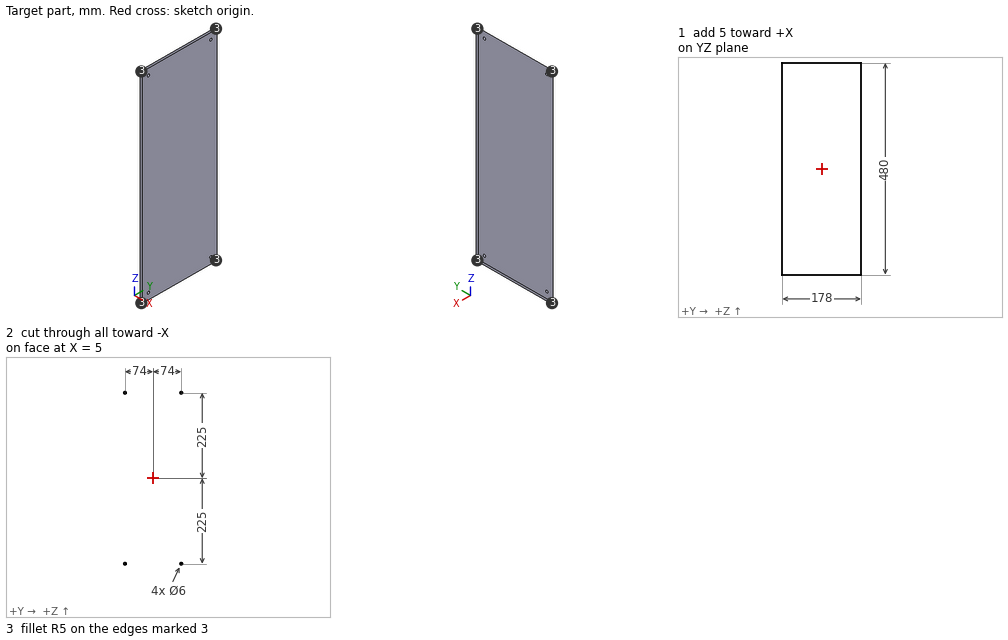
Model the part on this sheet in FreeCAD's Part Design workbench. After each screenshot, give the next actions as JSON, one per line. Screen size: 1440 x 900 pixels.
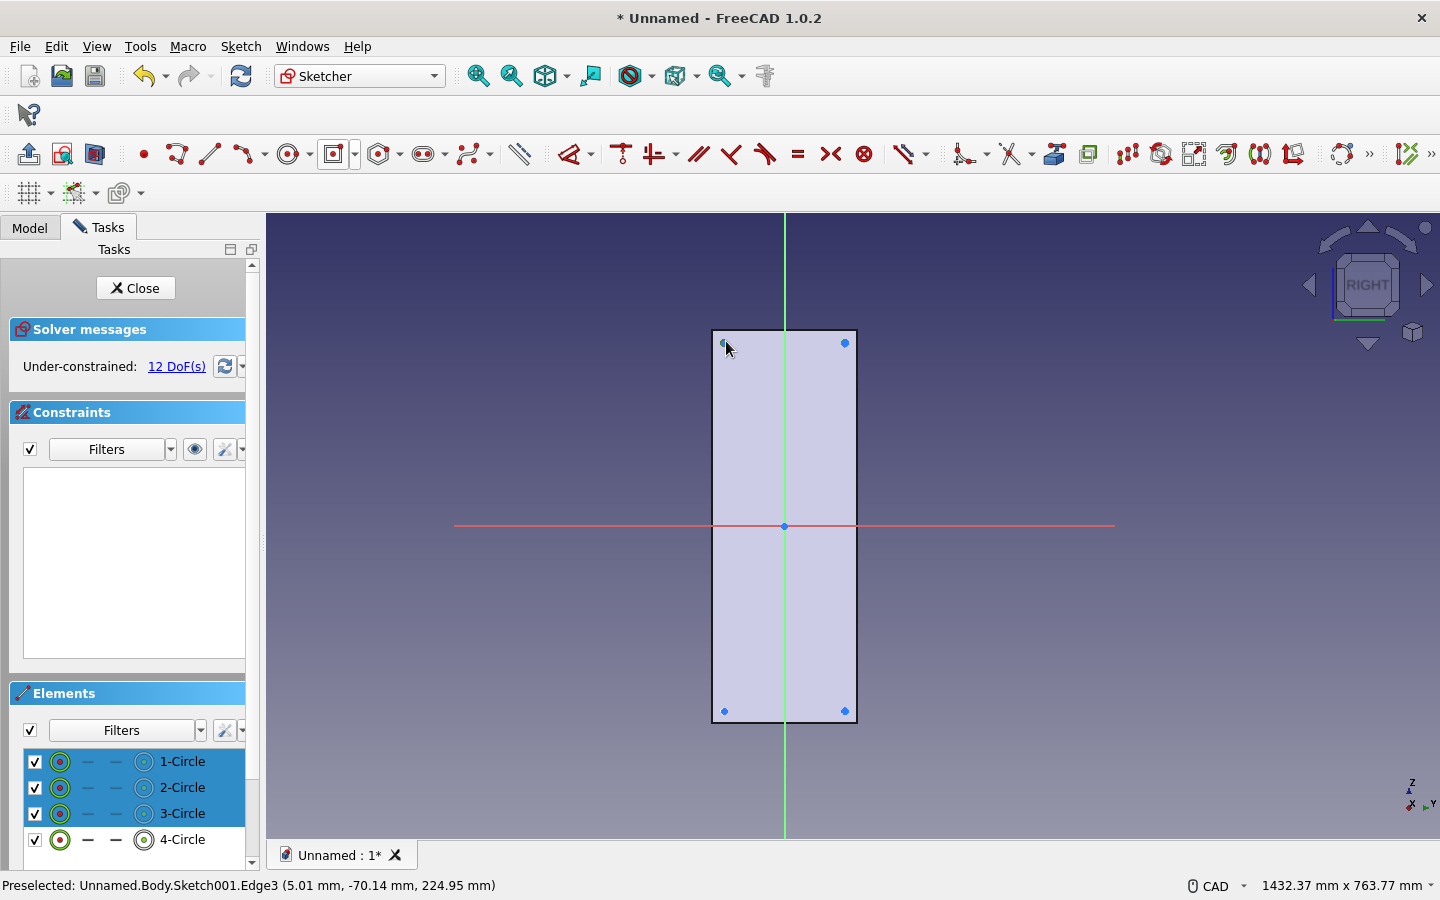
{"action": "scroll", "coordinate": [726, 709], "scroll_direction": "up", "scroll_amount": 9}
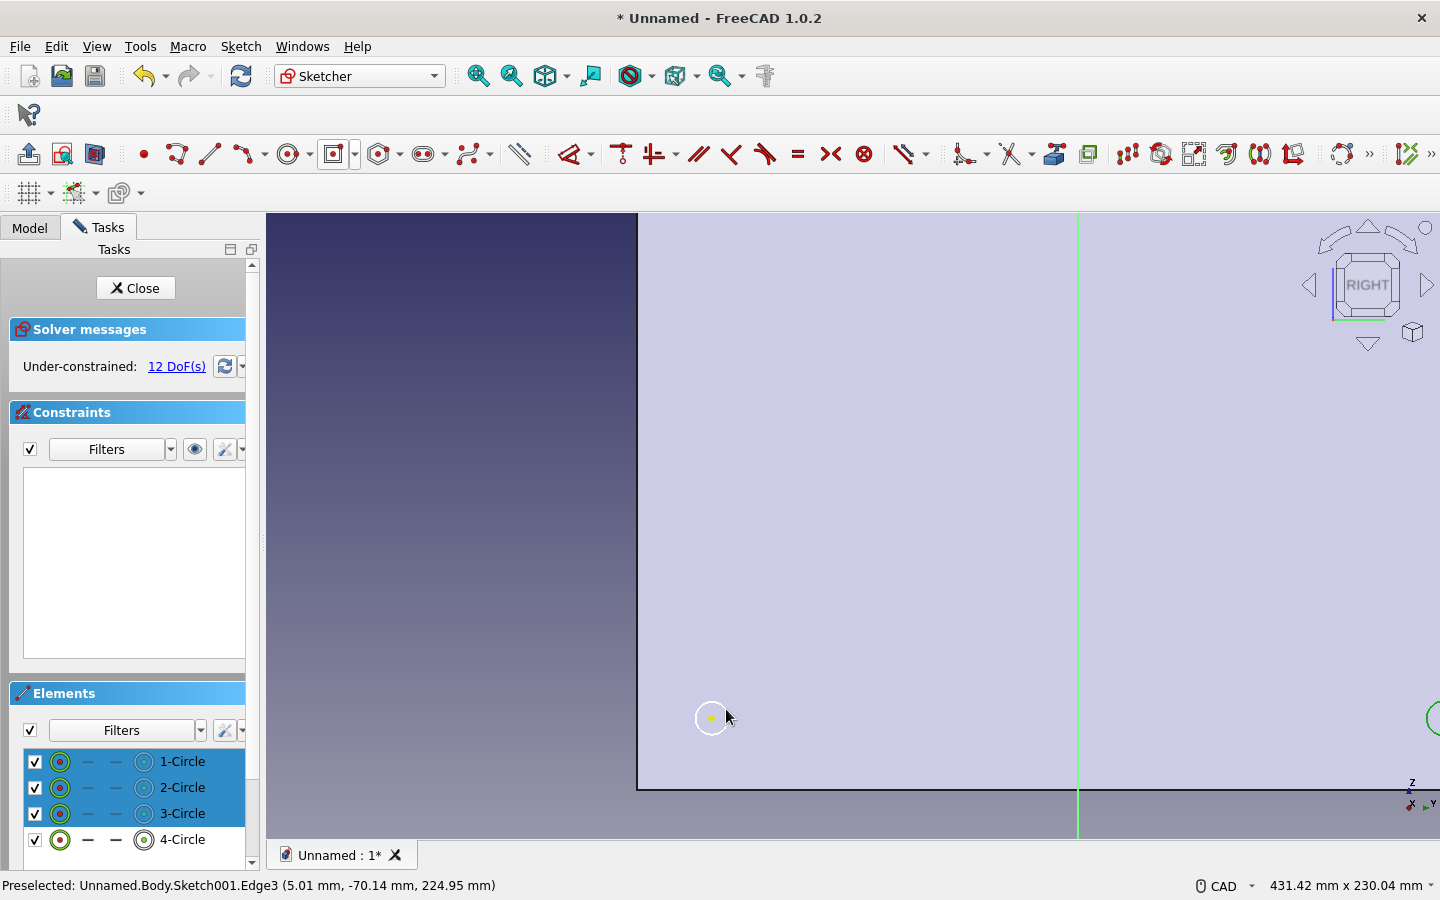
{"action": "left_click", "coordinate": [723, 707]}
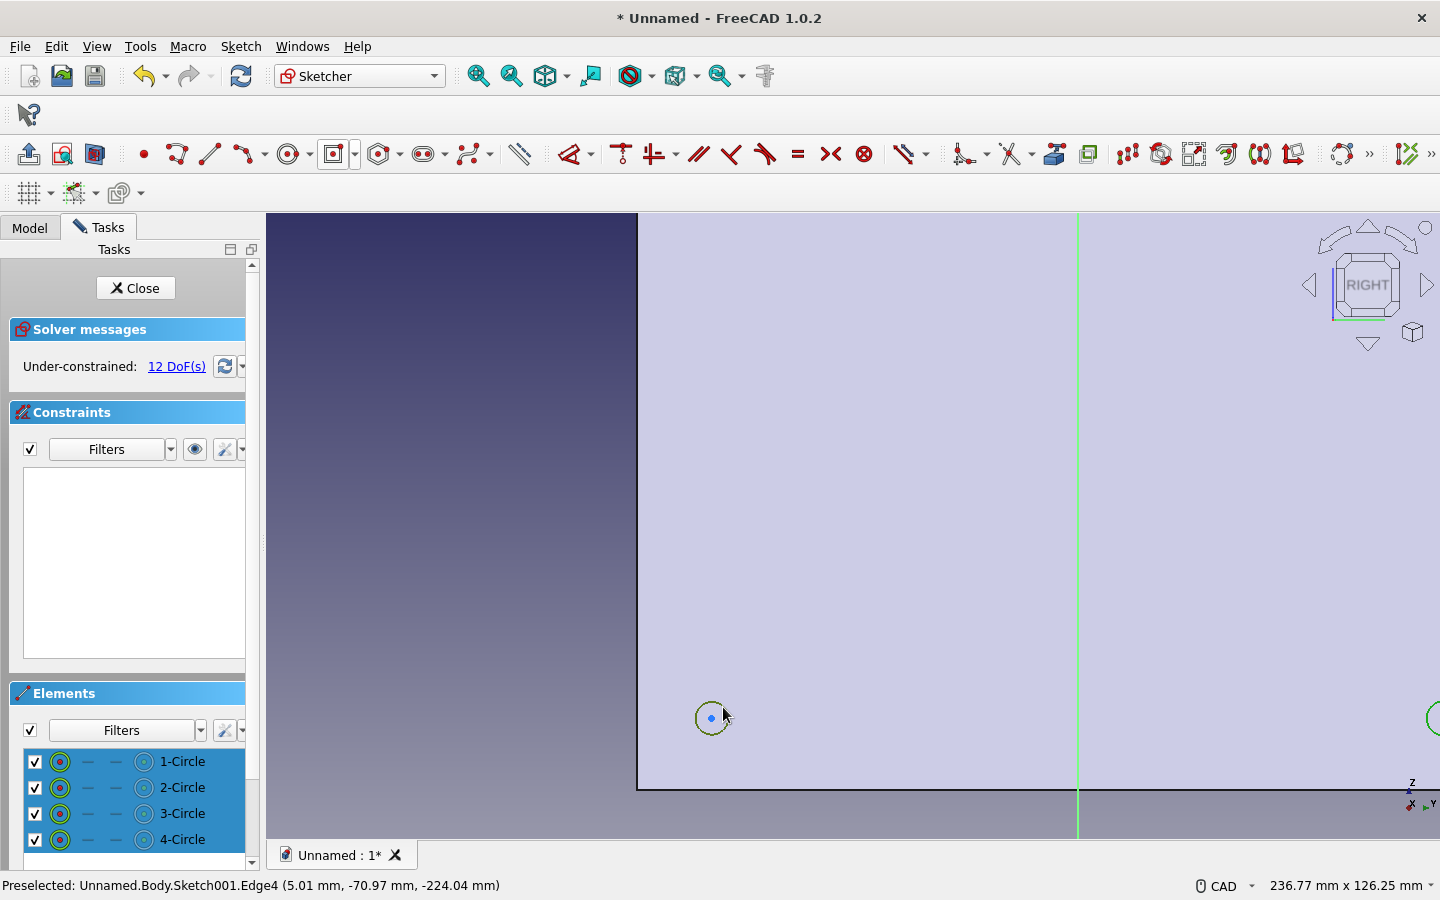
{"action": "left_click", "coordinate": [798, 154]}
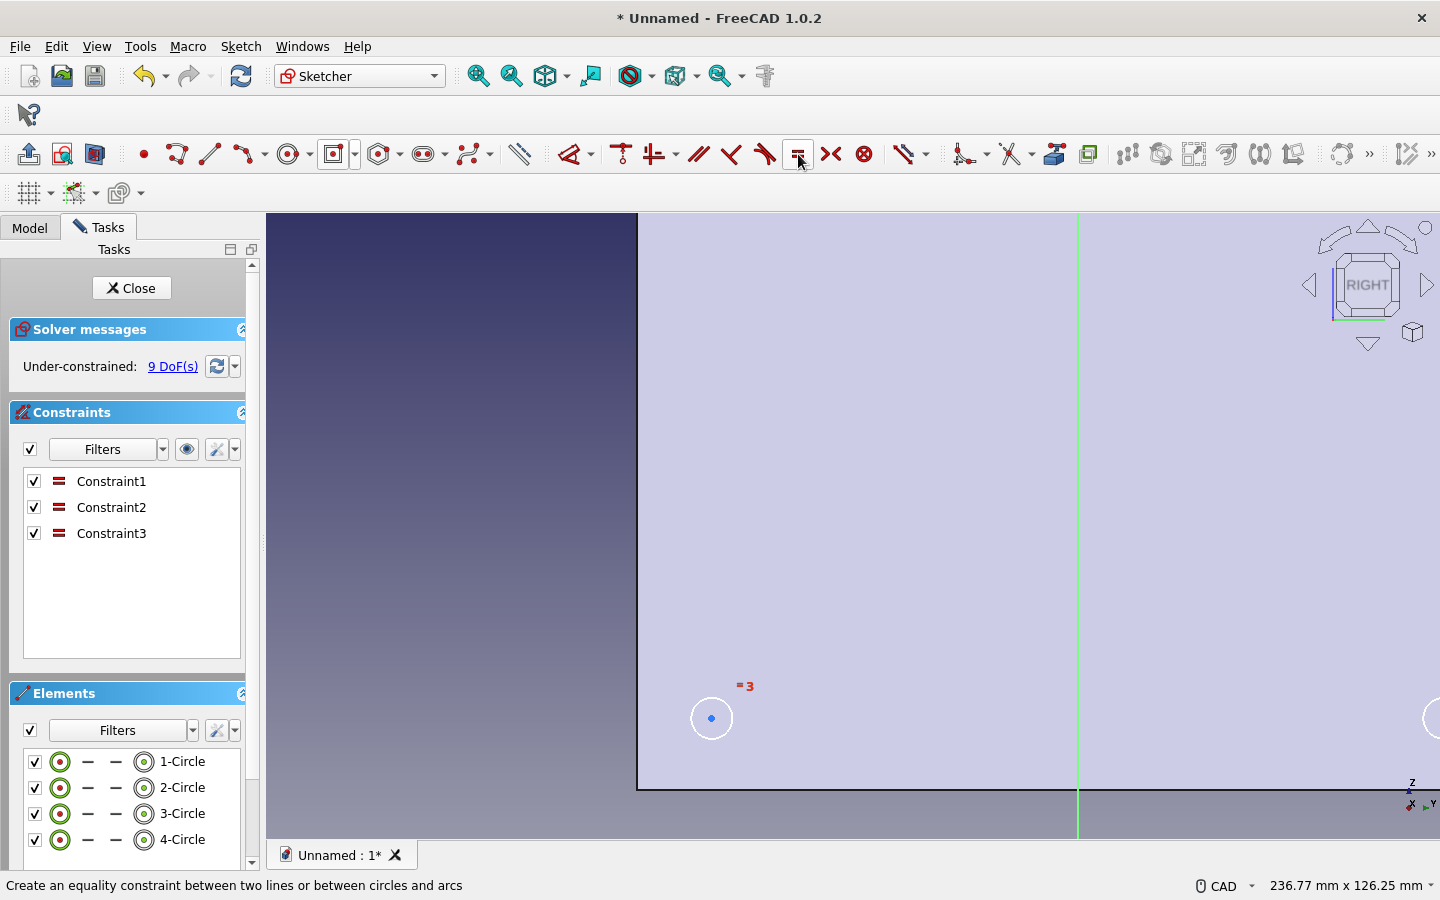
{"action": "scroll", "coordinate": [726, 709], "scroll_direction": "down", "scroll_amount": 9}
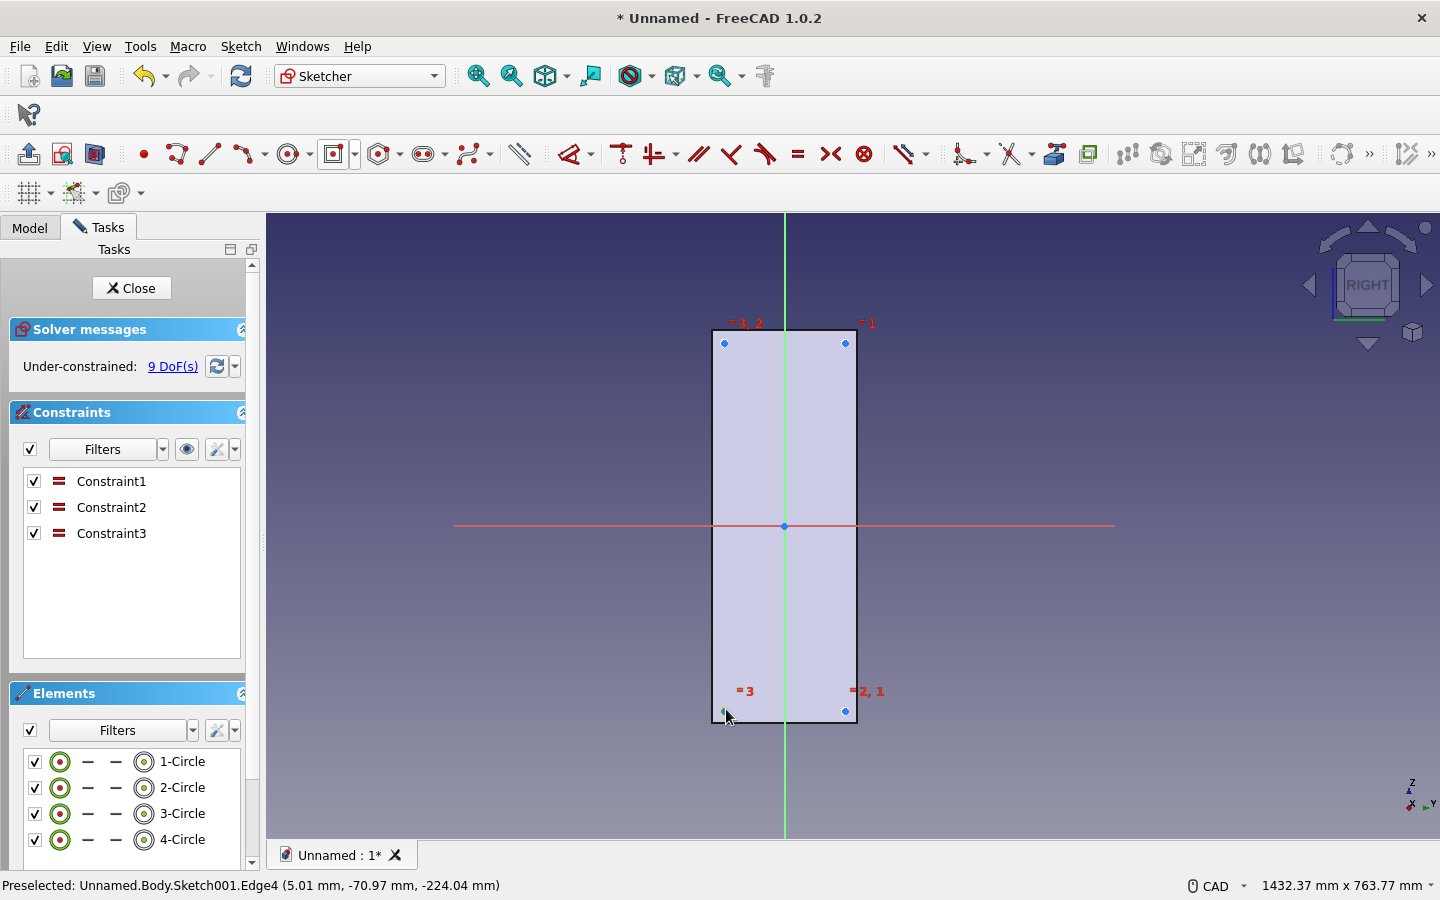
{"action": "left_click", "coordinate": [845, 343]}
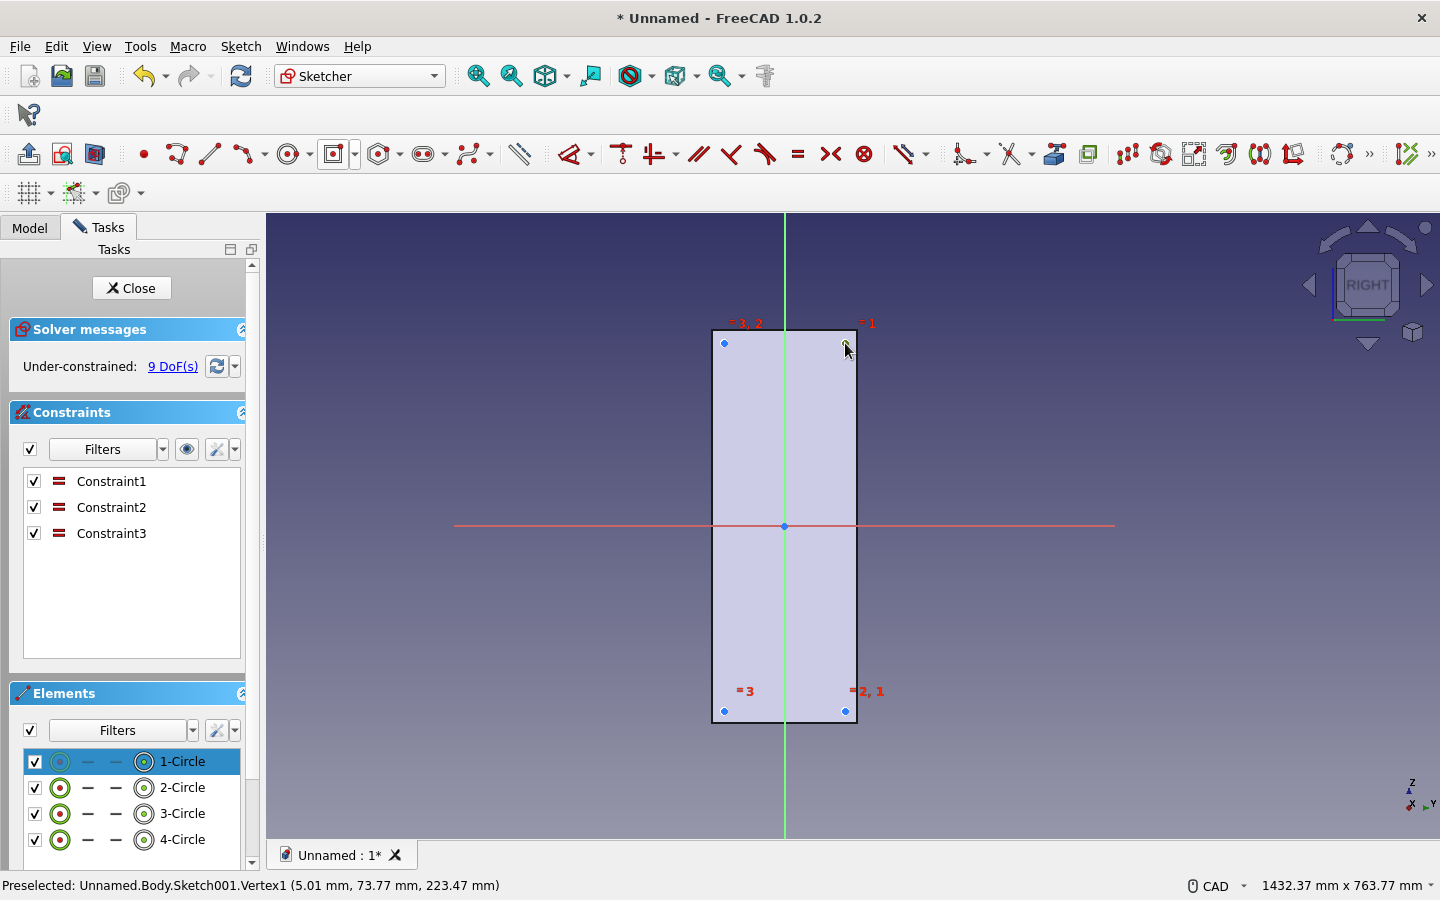
{"action": "left_click", "coordinate": [845, 711]}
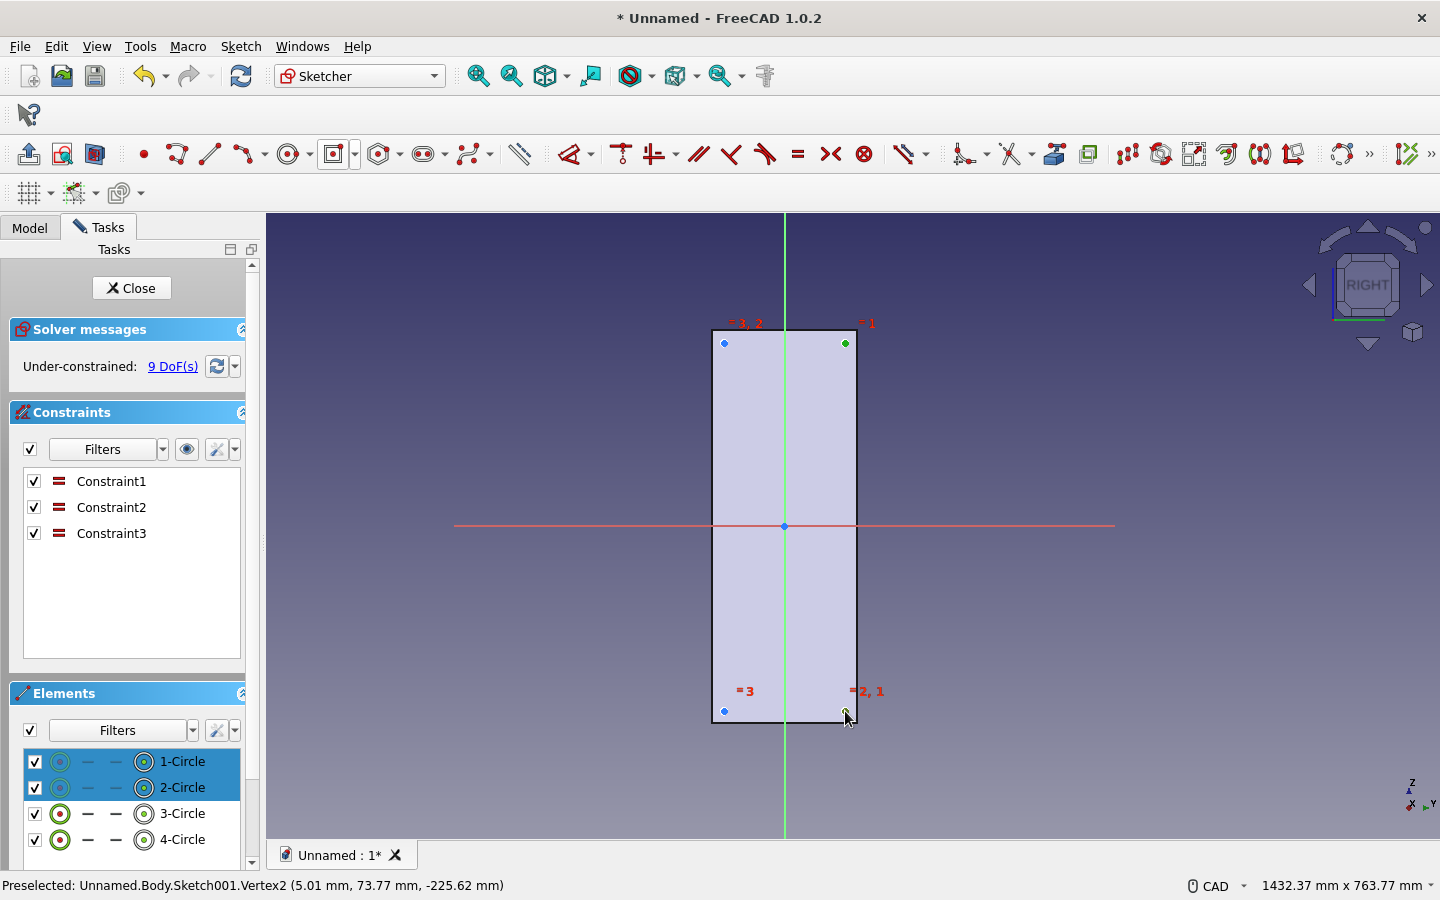
{"action": "key", "text": "v"}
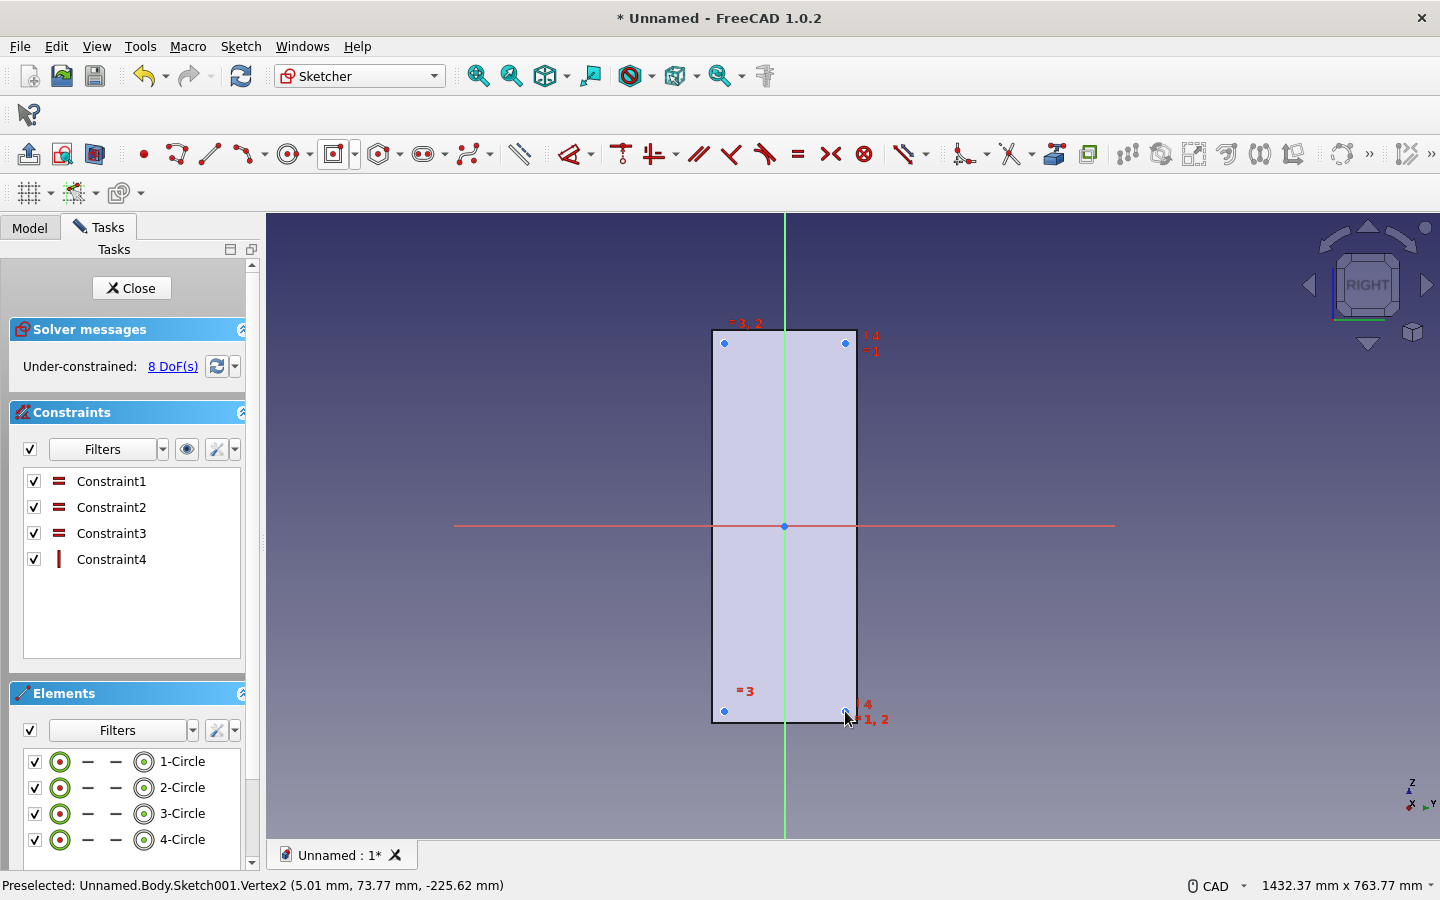
{"action": "left_click", "coordinate": [845, 343]}